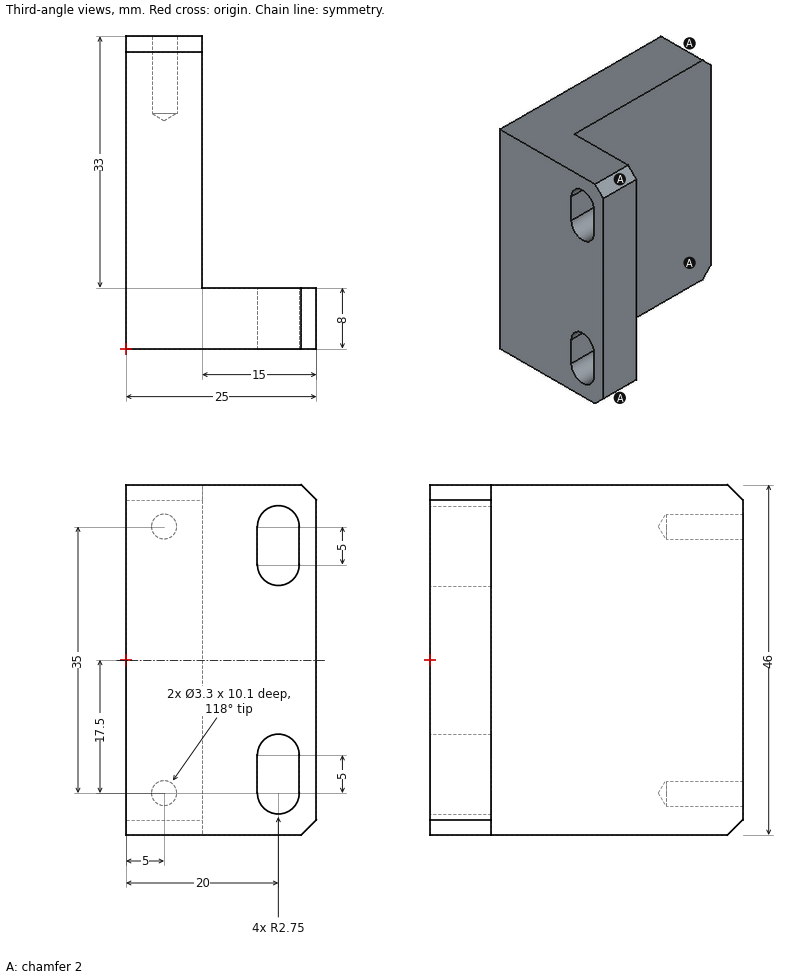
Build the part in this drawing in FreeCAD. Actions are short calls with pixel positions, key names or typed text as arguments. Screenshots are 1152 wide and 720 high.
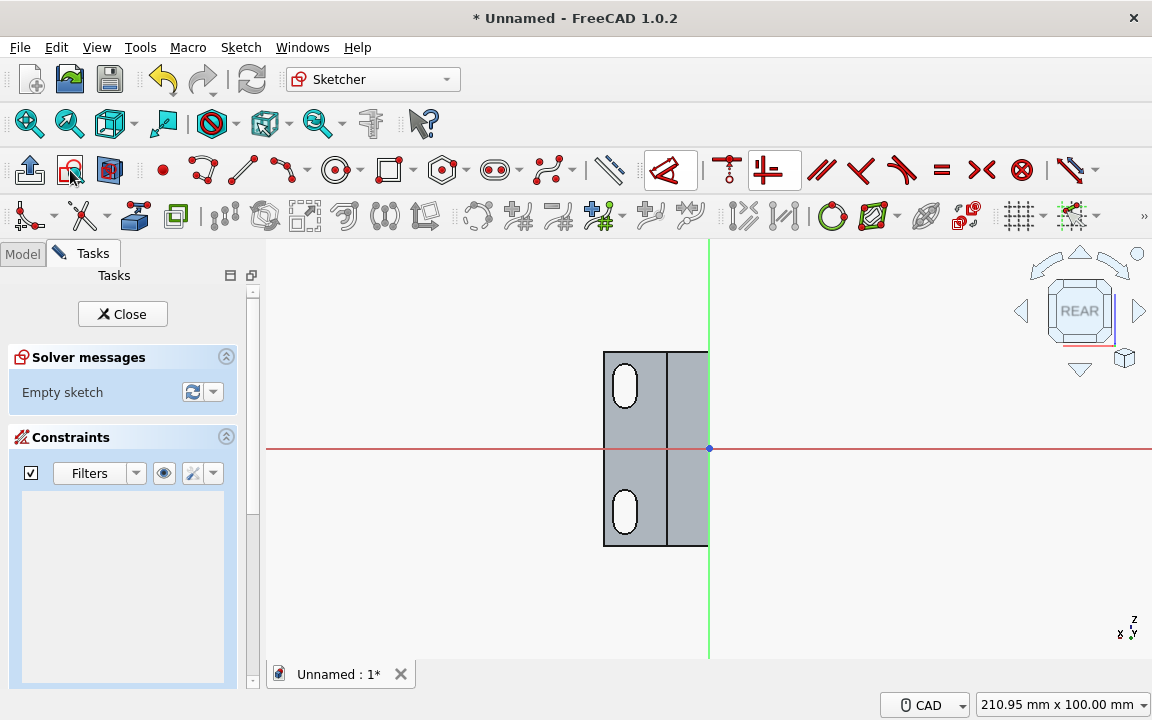
scroll(806, 449, up, 2)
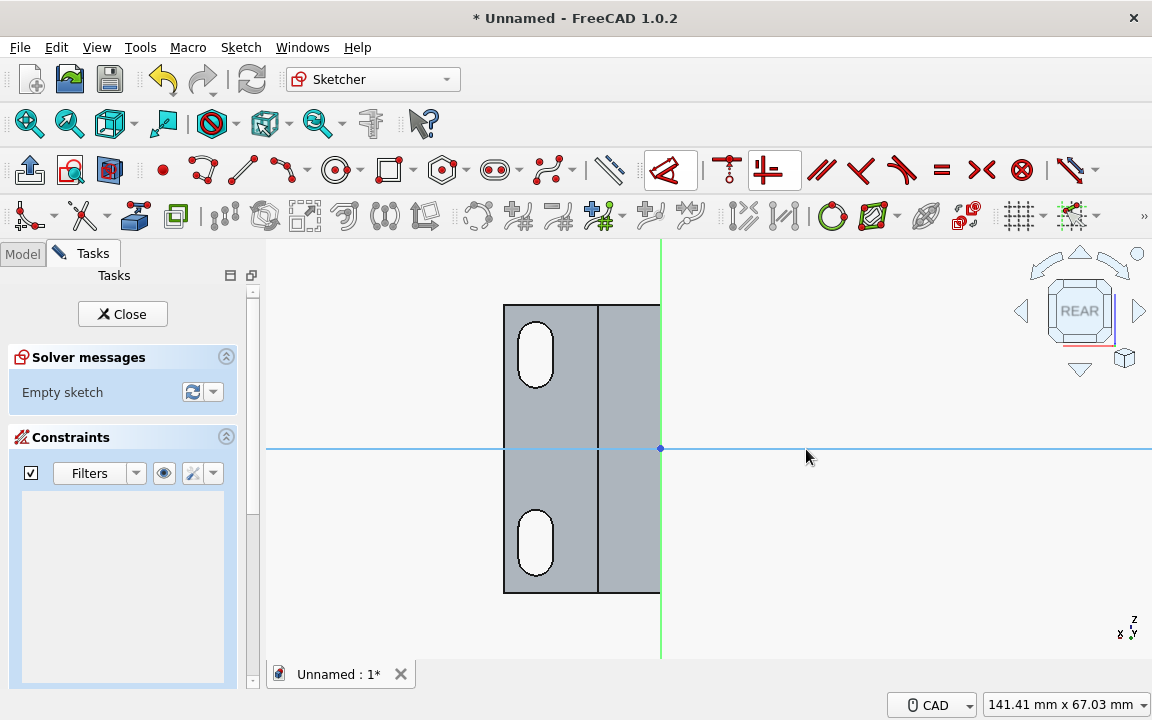
click(336, 170)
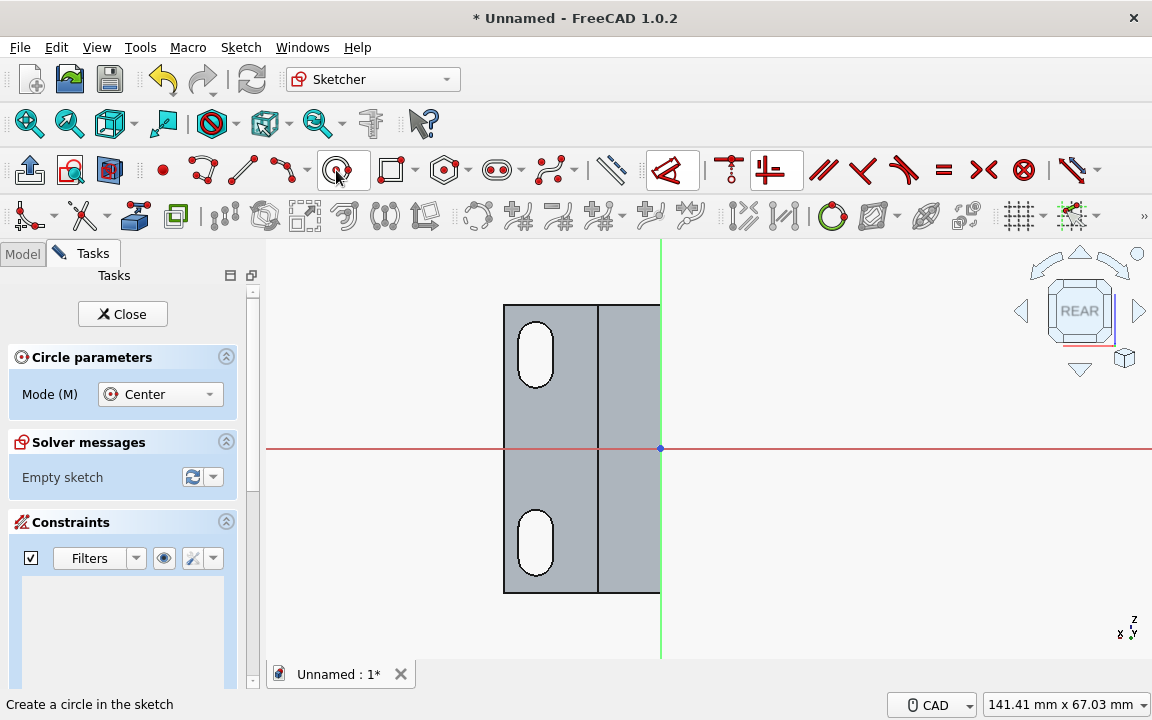
scroll(630, 558, up, 4)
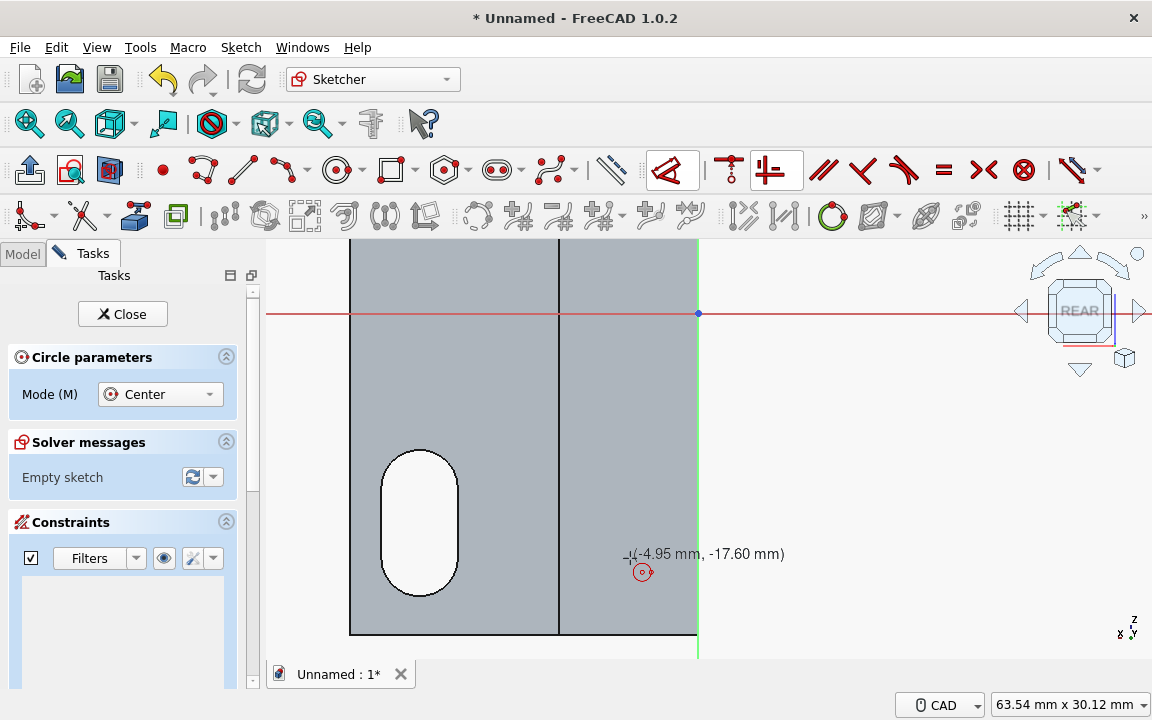
click(629, 558)
click(645, 542)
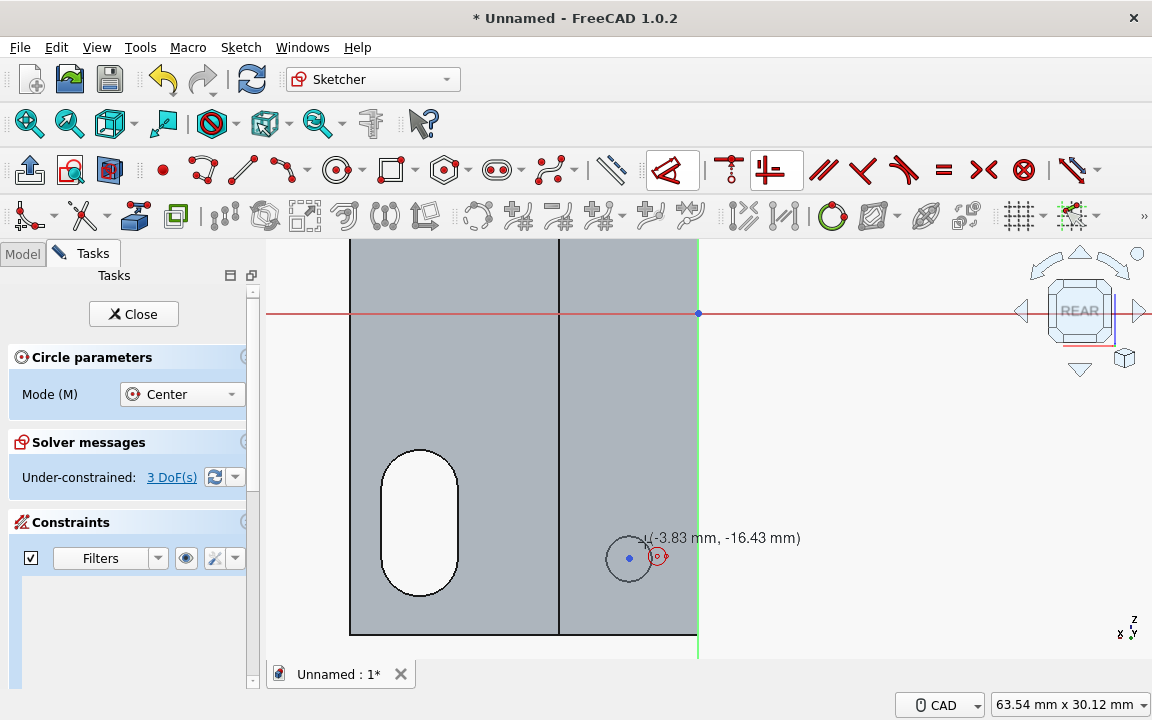
scroll(631, 559, down, 4)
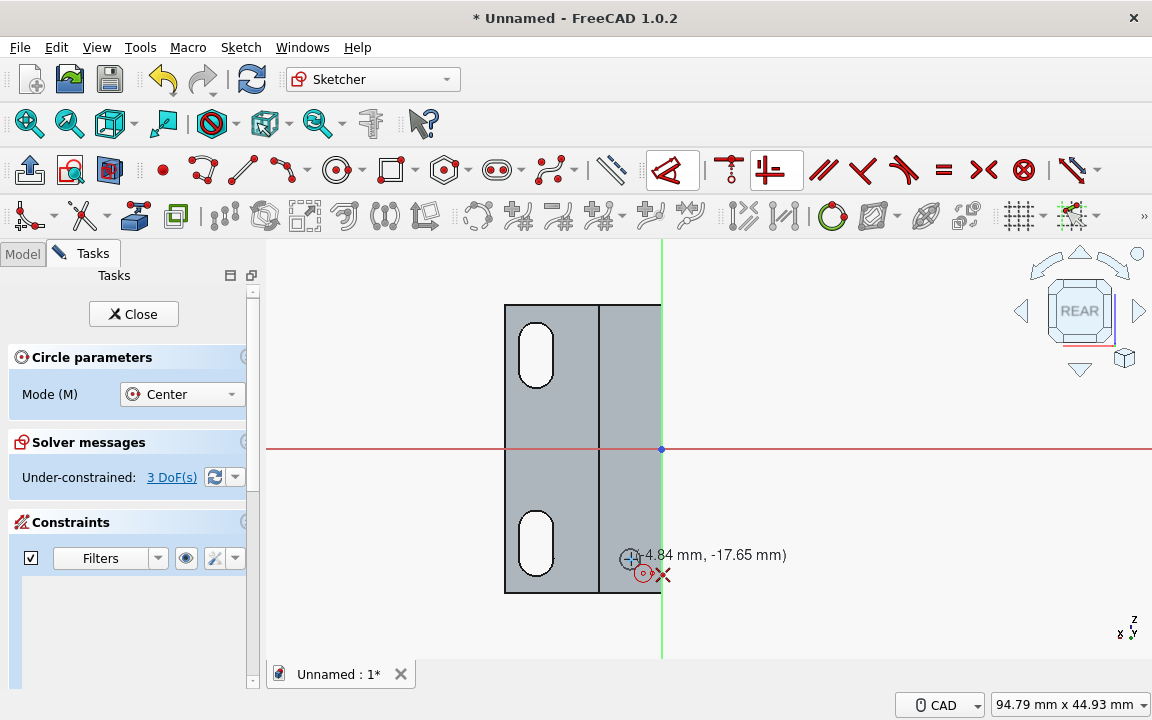
scroll(630, 340, up, 4)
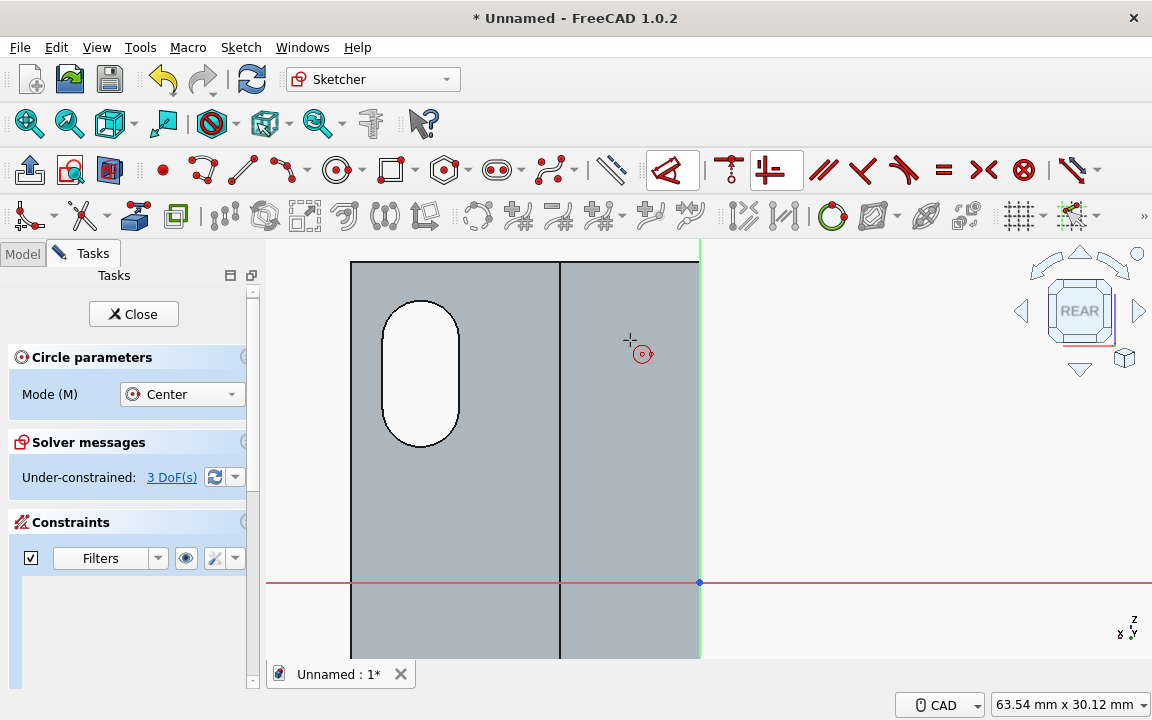
click(630, 339)
click(646, 323)
key(Escape)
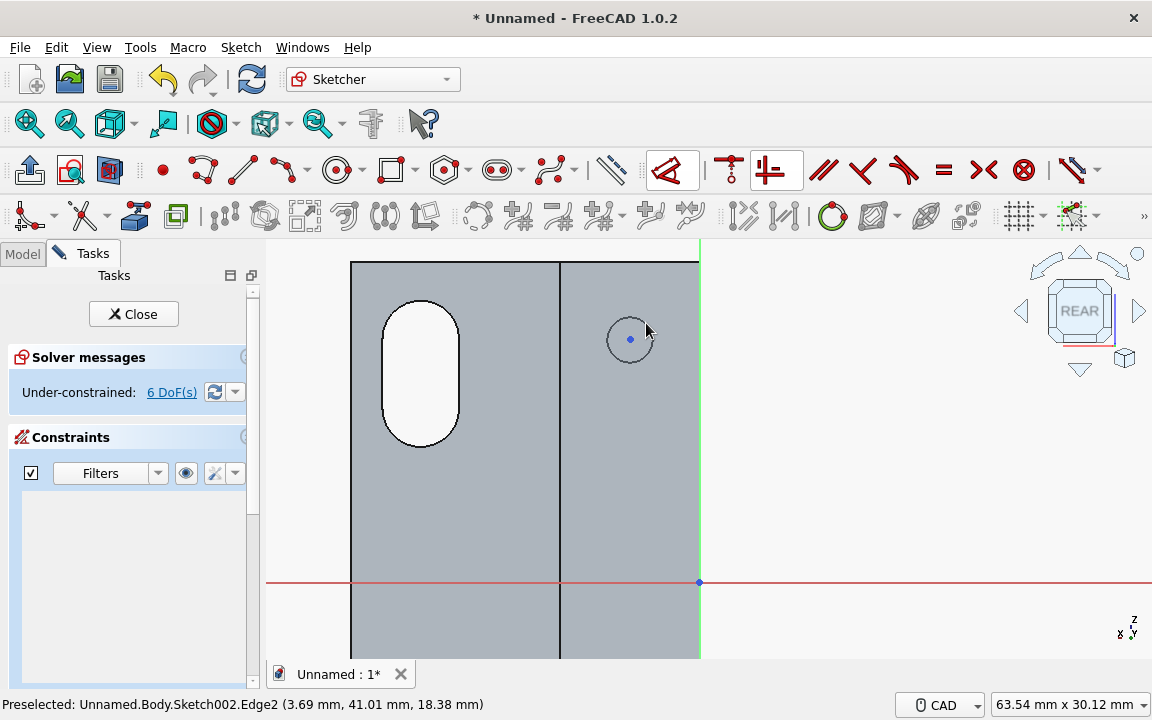
scroll(630, 340, down, 4)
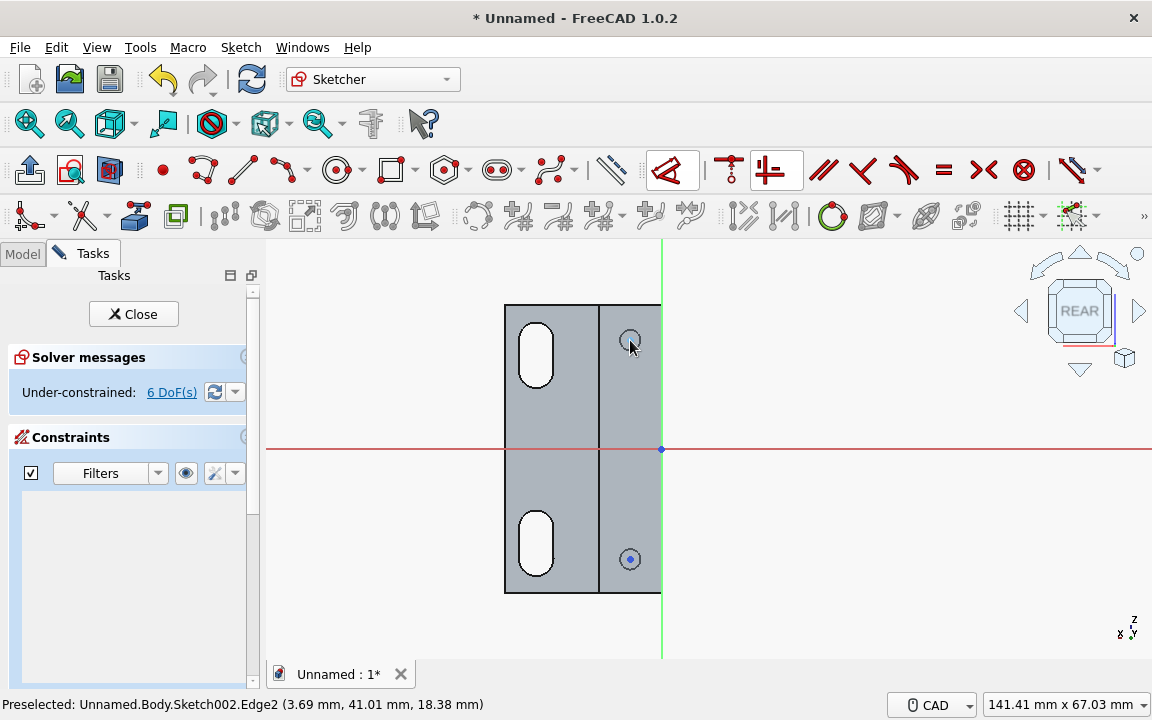
scroll(637, 552, up, 2)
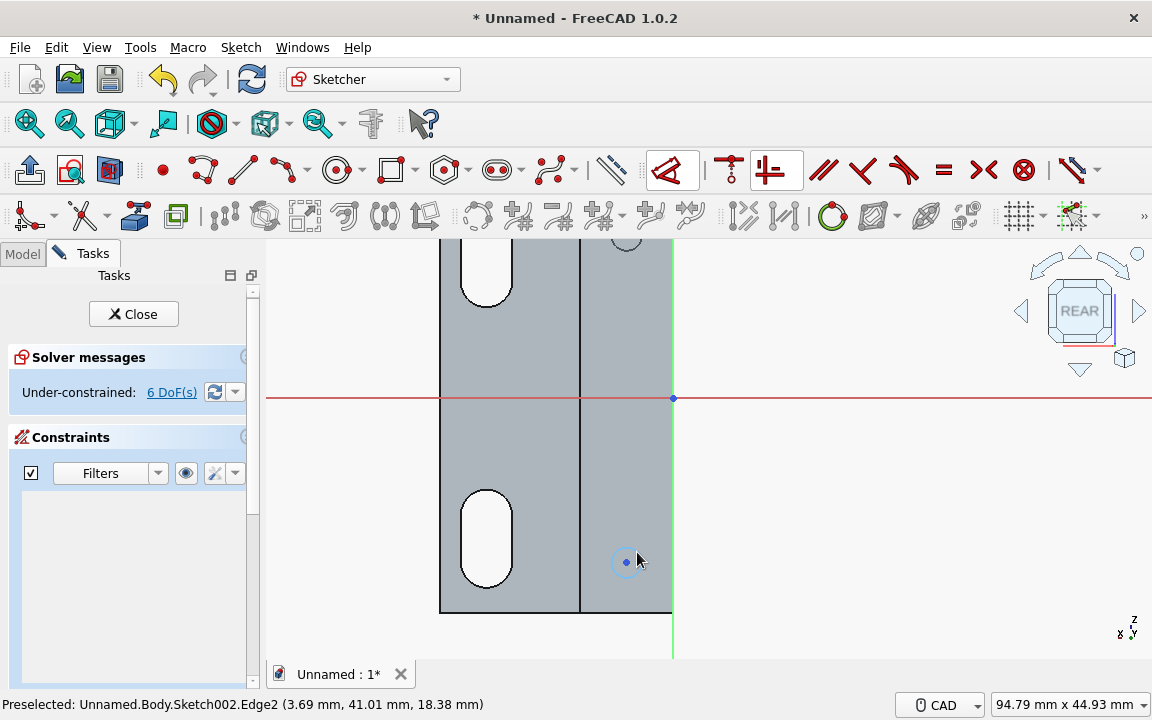
click(638, 552)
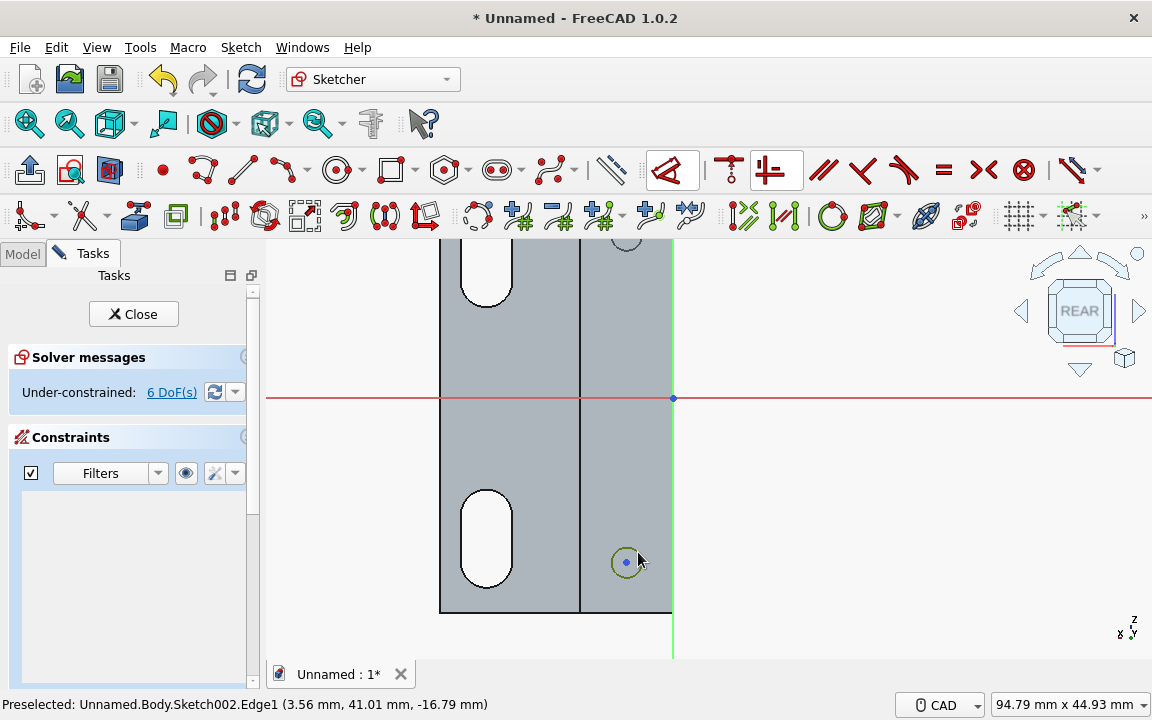
scroll(637, 552, down, 2)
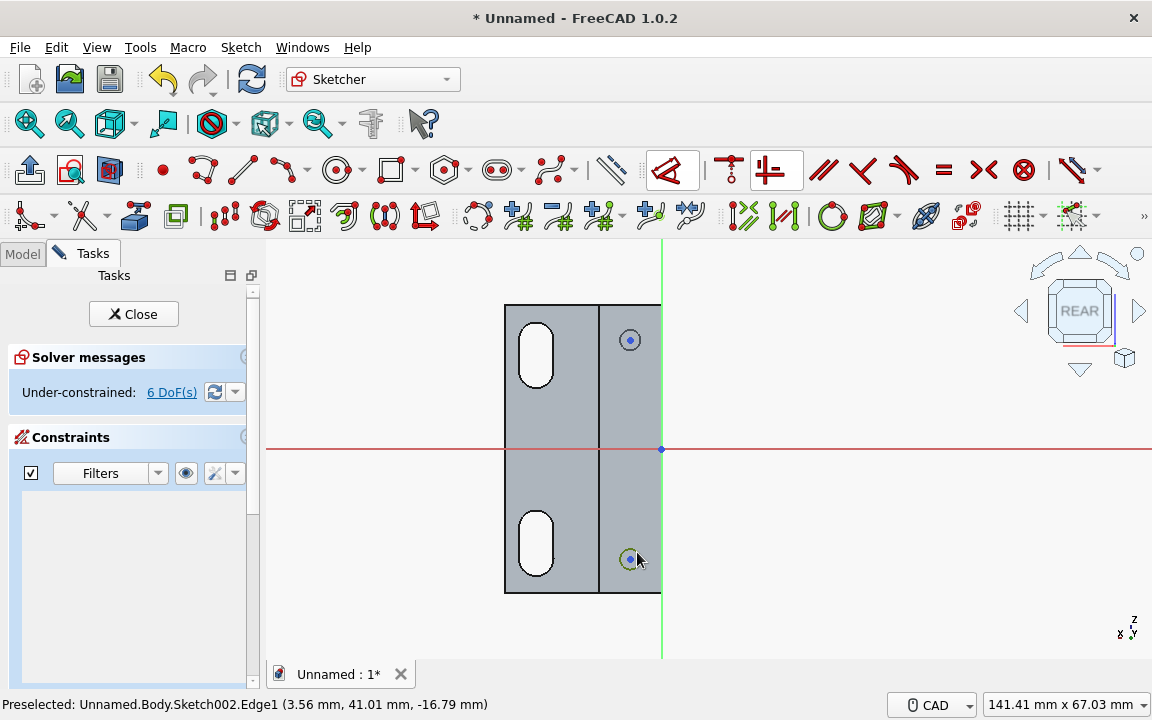
scroll(637, 333, up, 2)